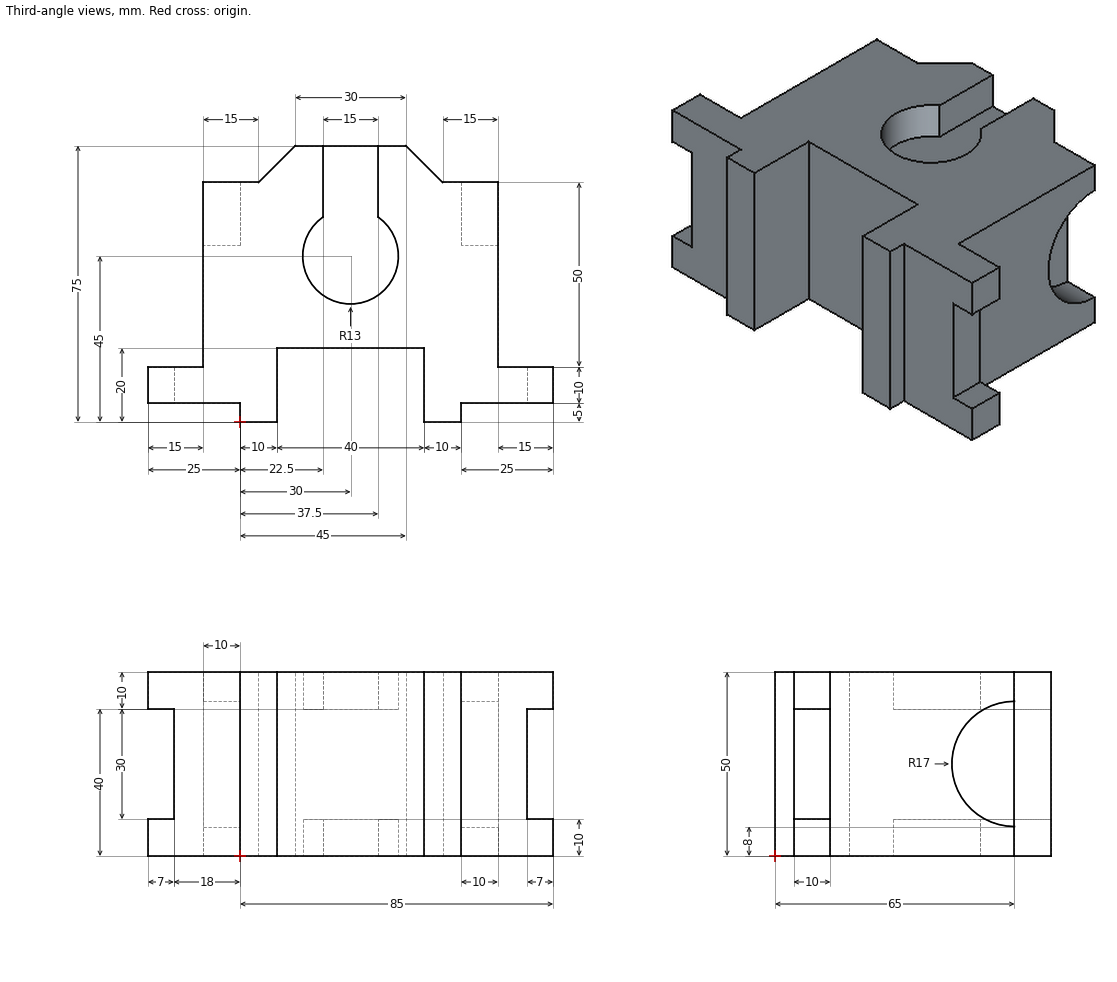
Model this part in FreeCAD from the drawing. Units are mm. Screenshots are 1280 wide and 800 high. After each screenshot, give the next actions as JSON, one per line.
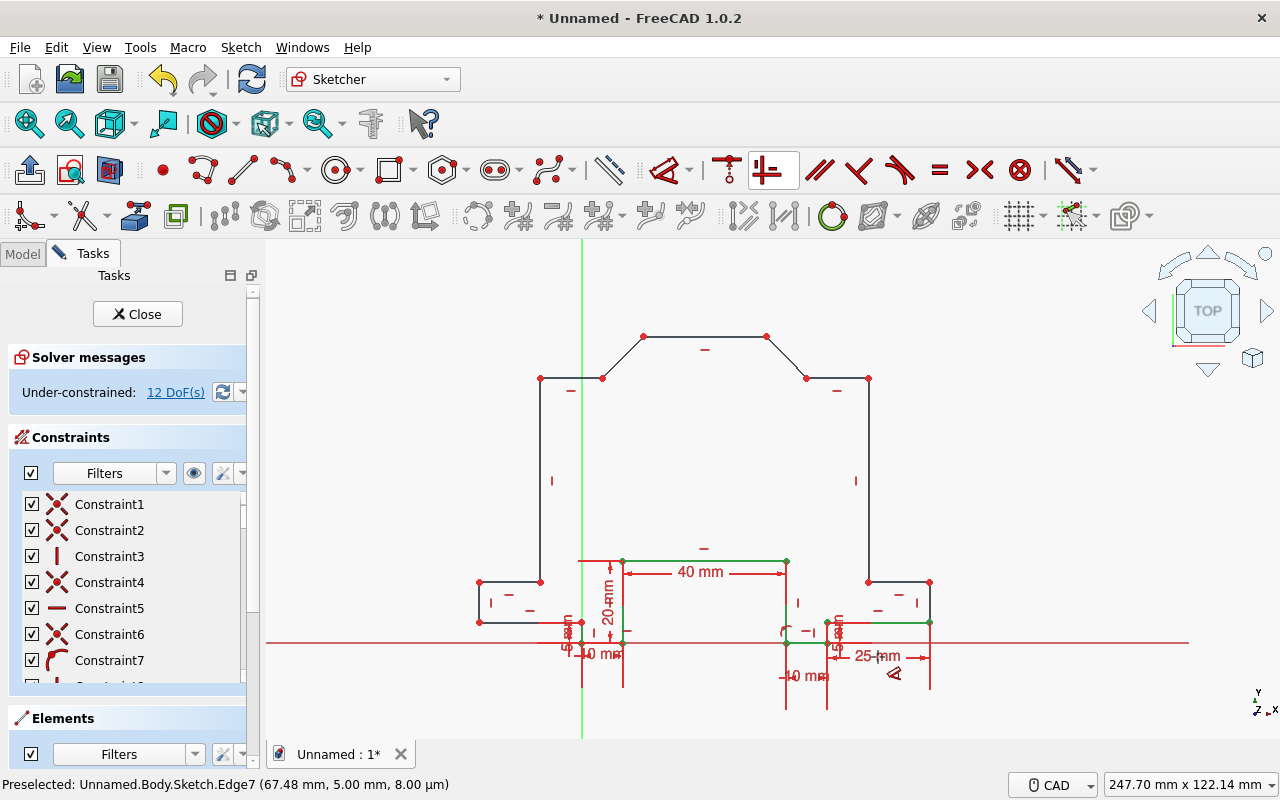
{"action": "left_click", "coordinate": [930, 610]}
{"action": "left_click", "coordinate": [964, 602]}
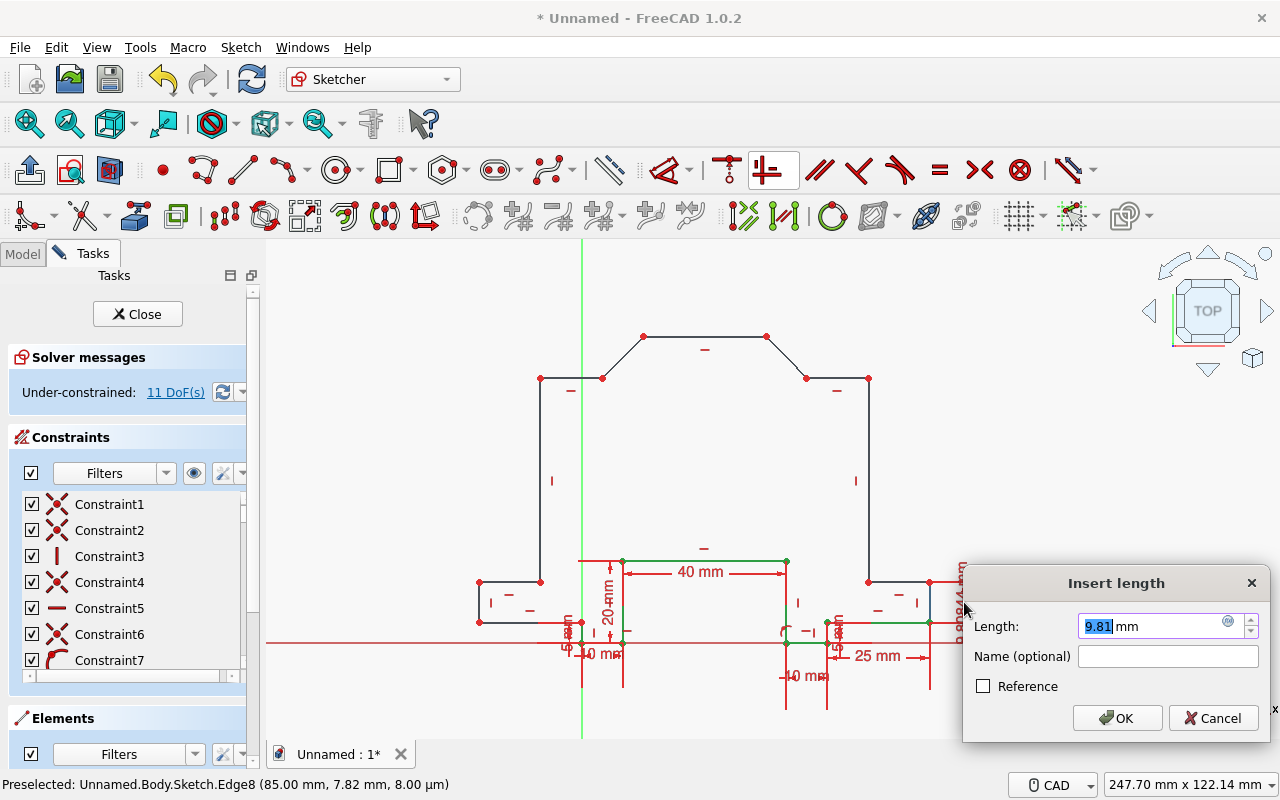
{"action": "type", "text": "10"}
{"action": "key", "text": "Return"}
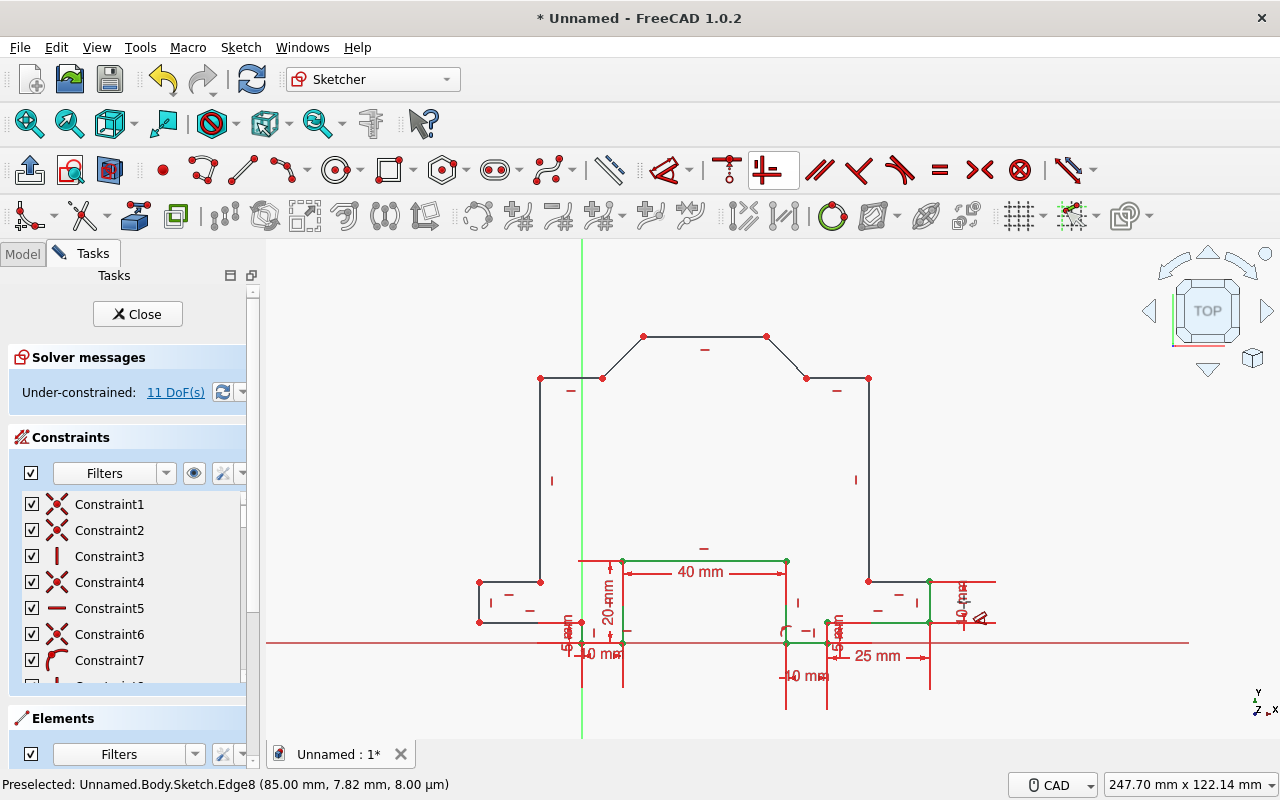
{"action": "left_click", "coordinate": [911, 582]}
{"action": "left_click", "coordinate": [899, 548]}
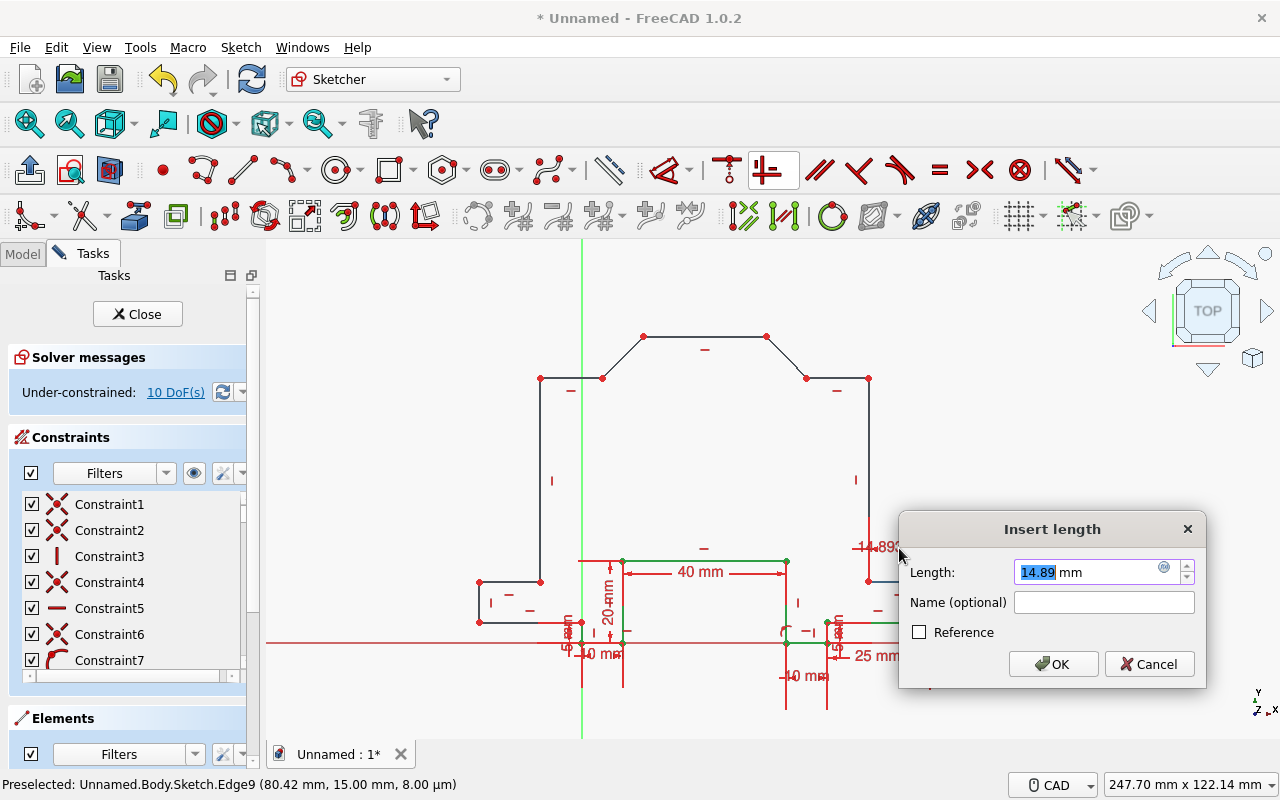
{"action": "type", "text": "15"}
{"action": "key", "text": "Return"}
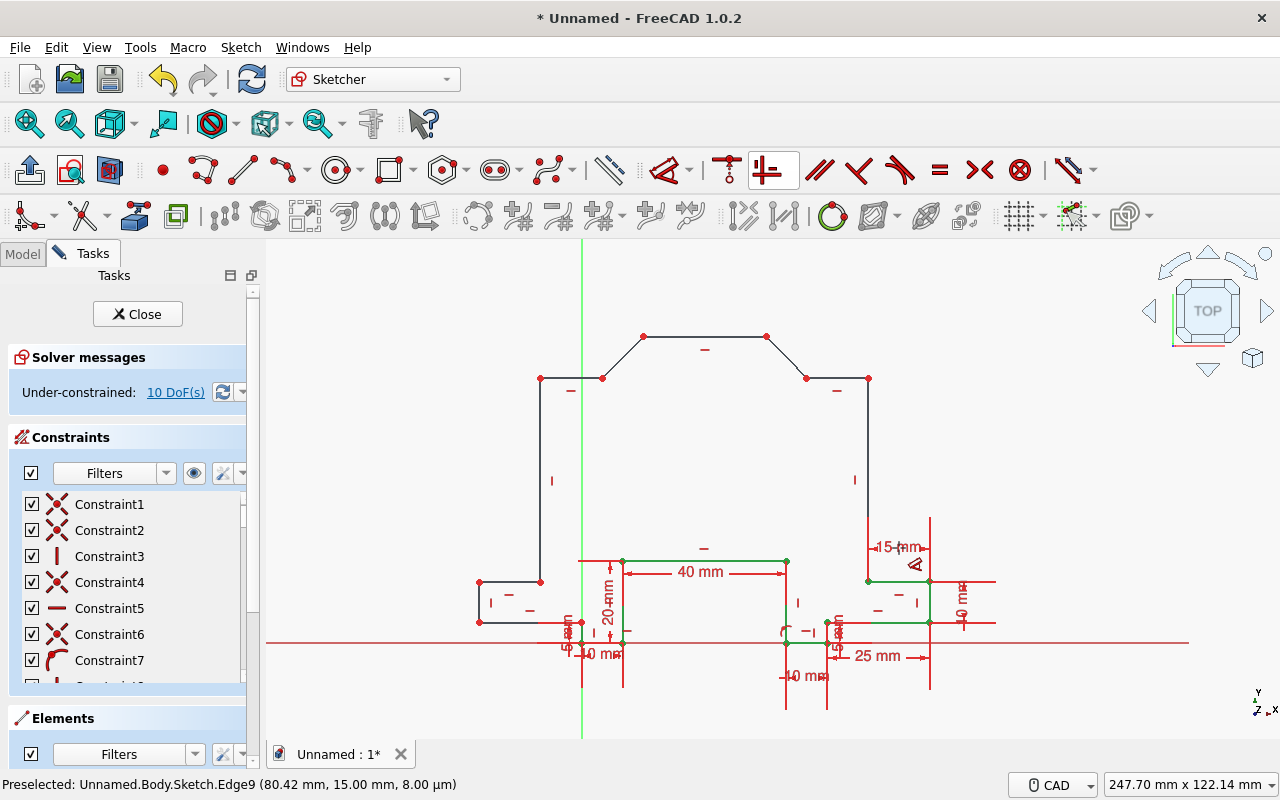
{"action": "left_click", "coordinate": [868, 521]}
{"action": "left_click", "coordinate": [902, 480]}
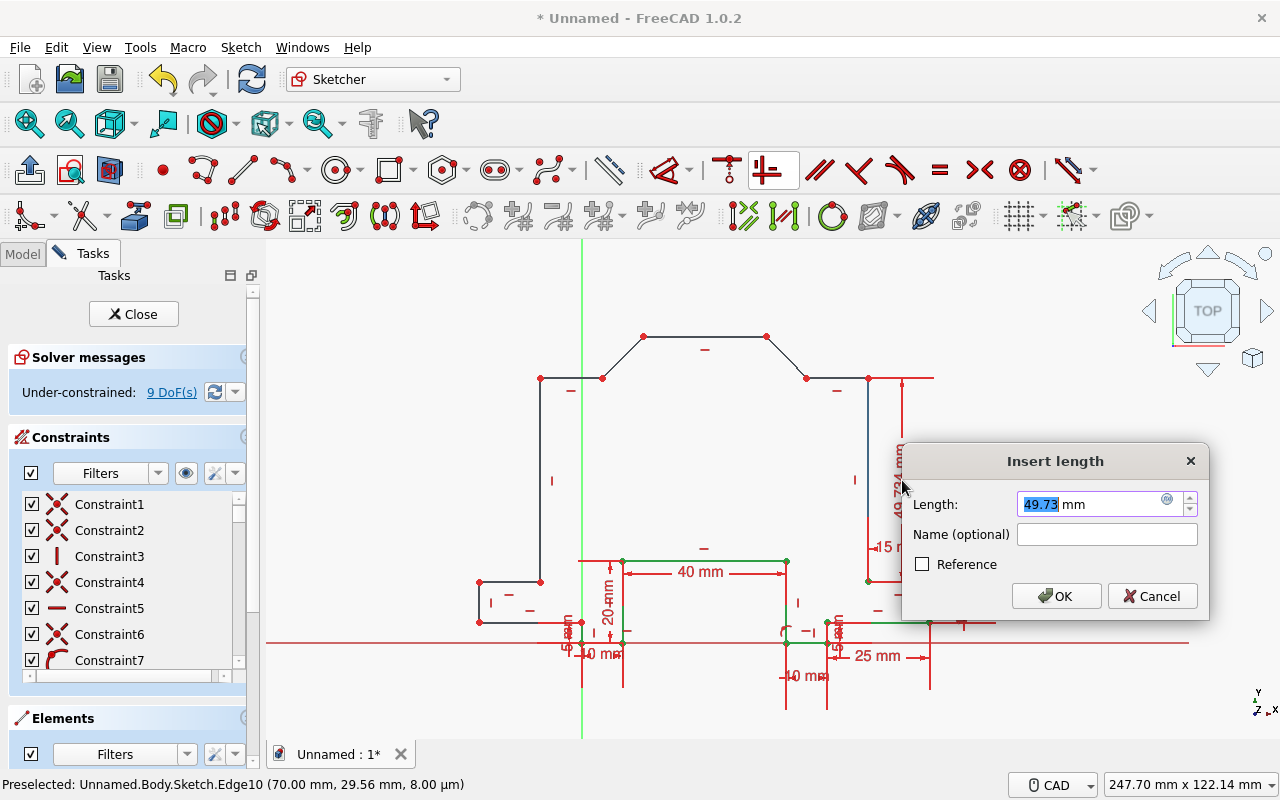
{"action": "type", "text": "50"}
{"action": "key", "text": "Return"}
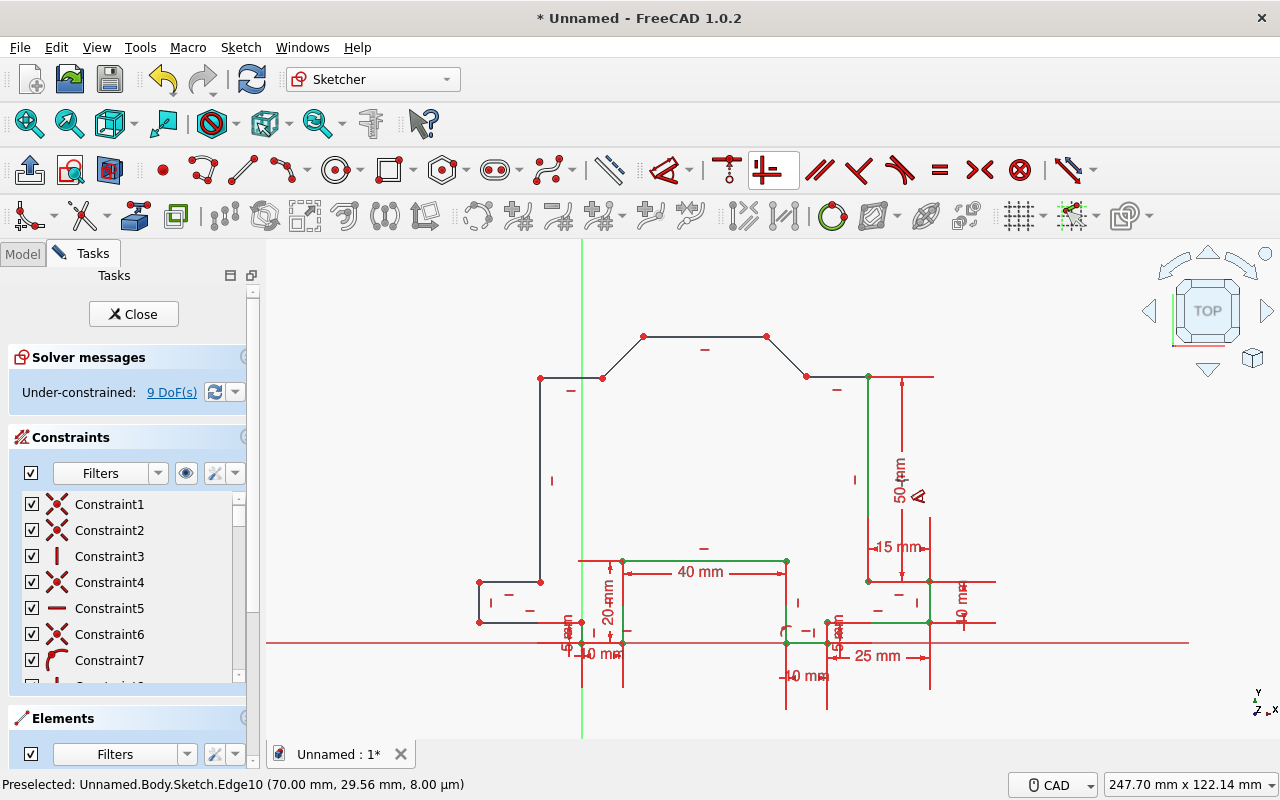
{"action": "left_click", "coordinate": [850, 377]}
{"action": "left_click", "coordinate": [838, 343]}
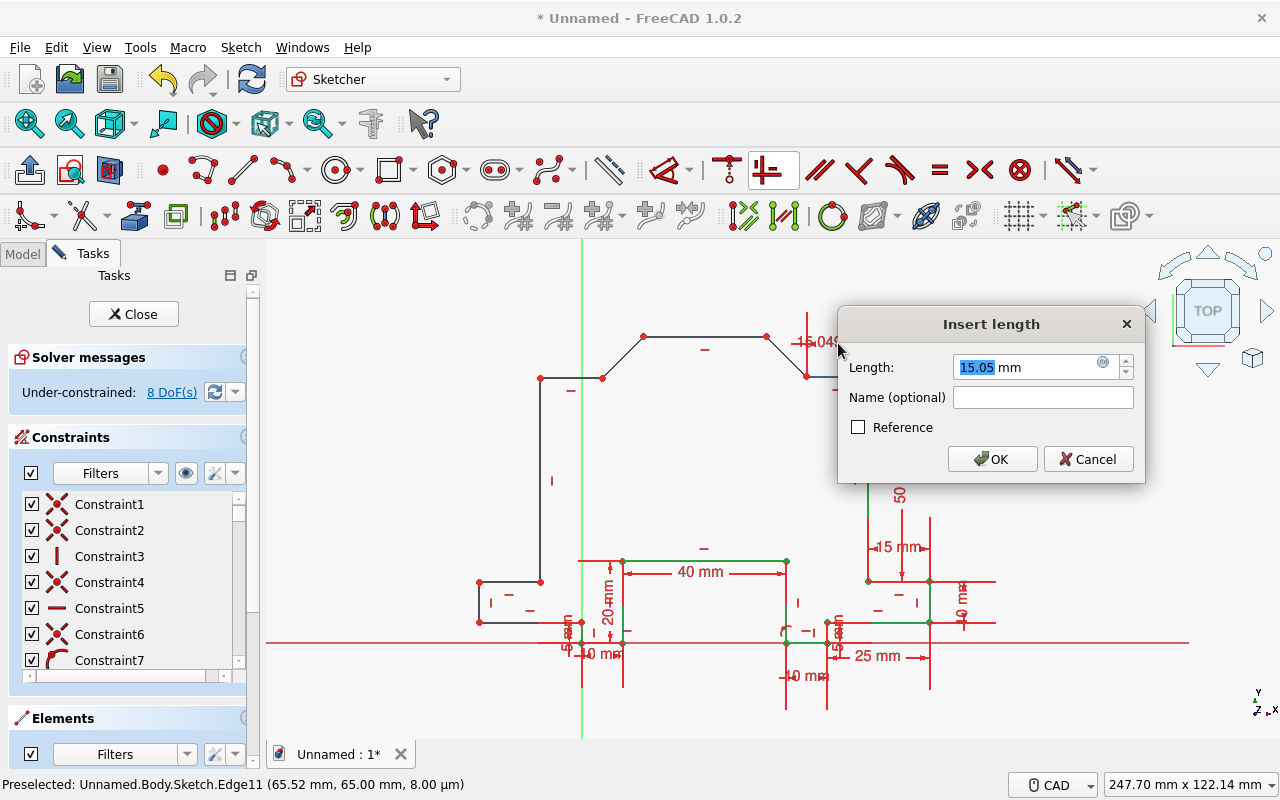
{"action": "type", "text": "15"}
{"action": "key", "text": "Return"}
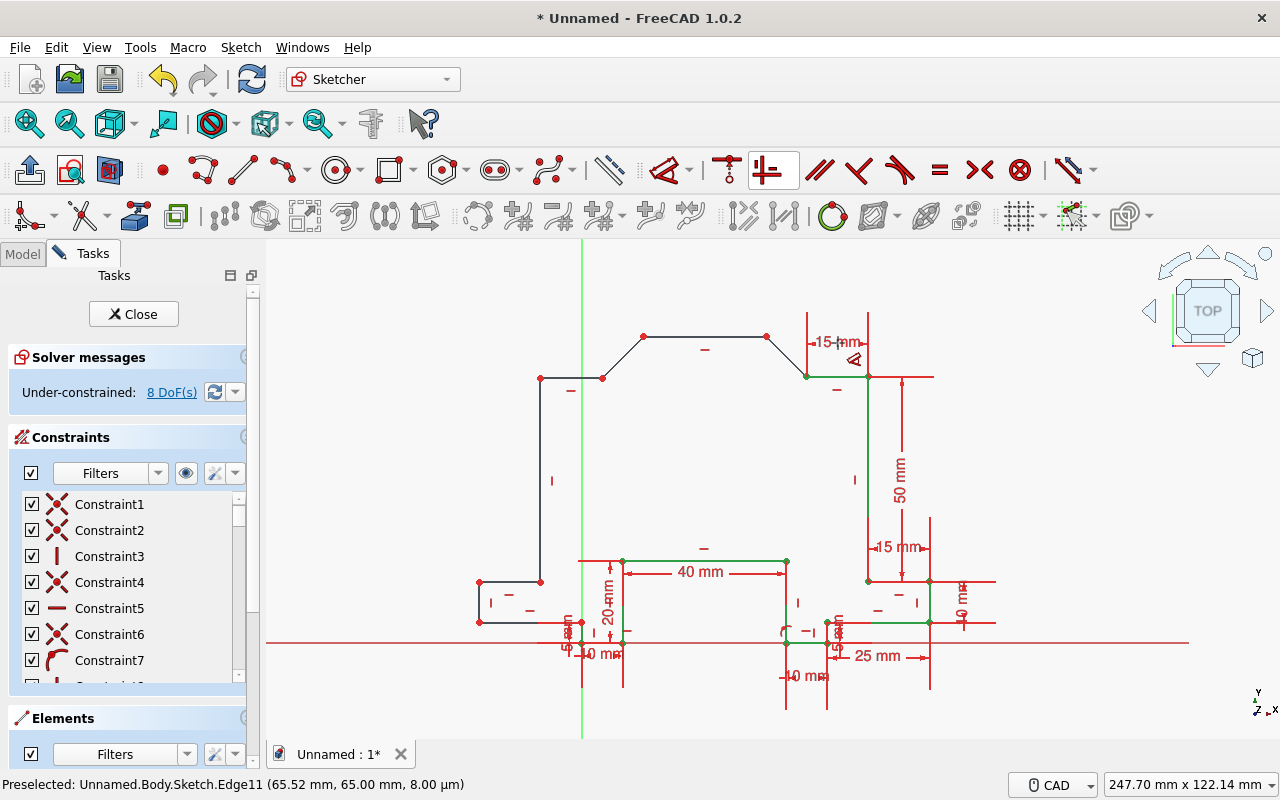
{"action": "left_click", "coordinate": [730, 337]}
{"action": "left_click", "coordinate": [705, 303]}